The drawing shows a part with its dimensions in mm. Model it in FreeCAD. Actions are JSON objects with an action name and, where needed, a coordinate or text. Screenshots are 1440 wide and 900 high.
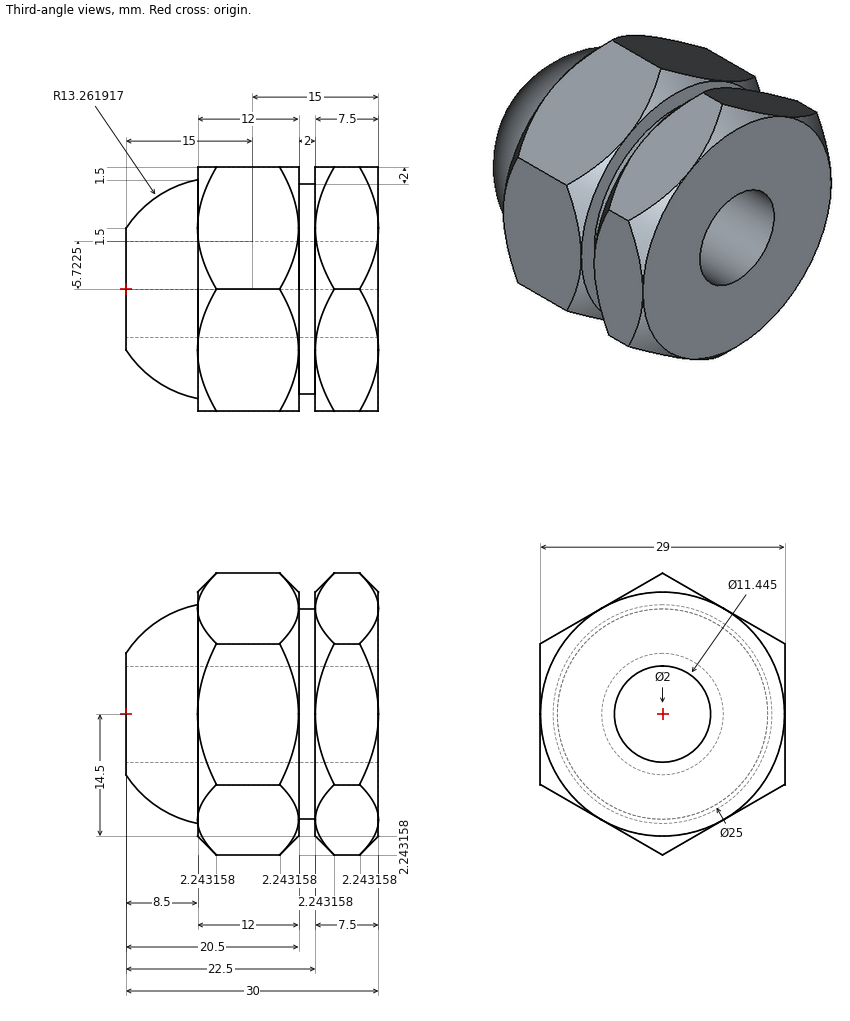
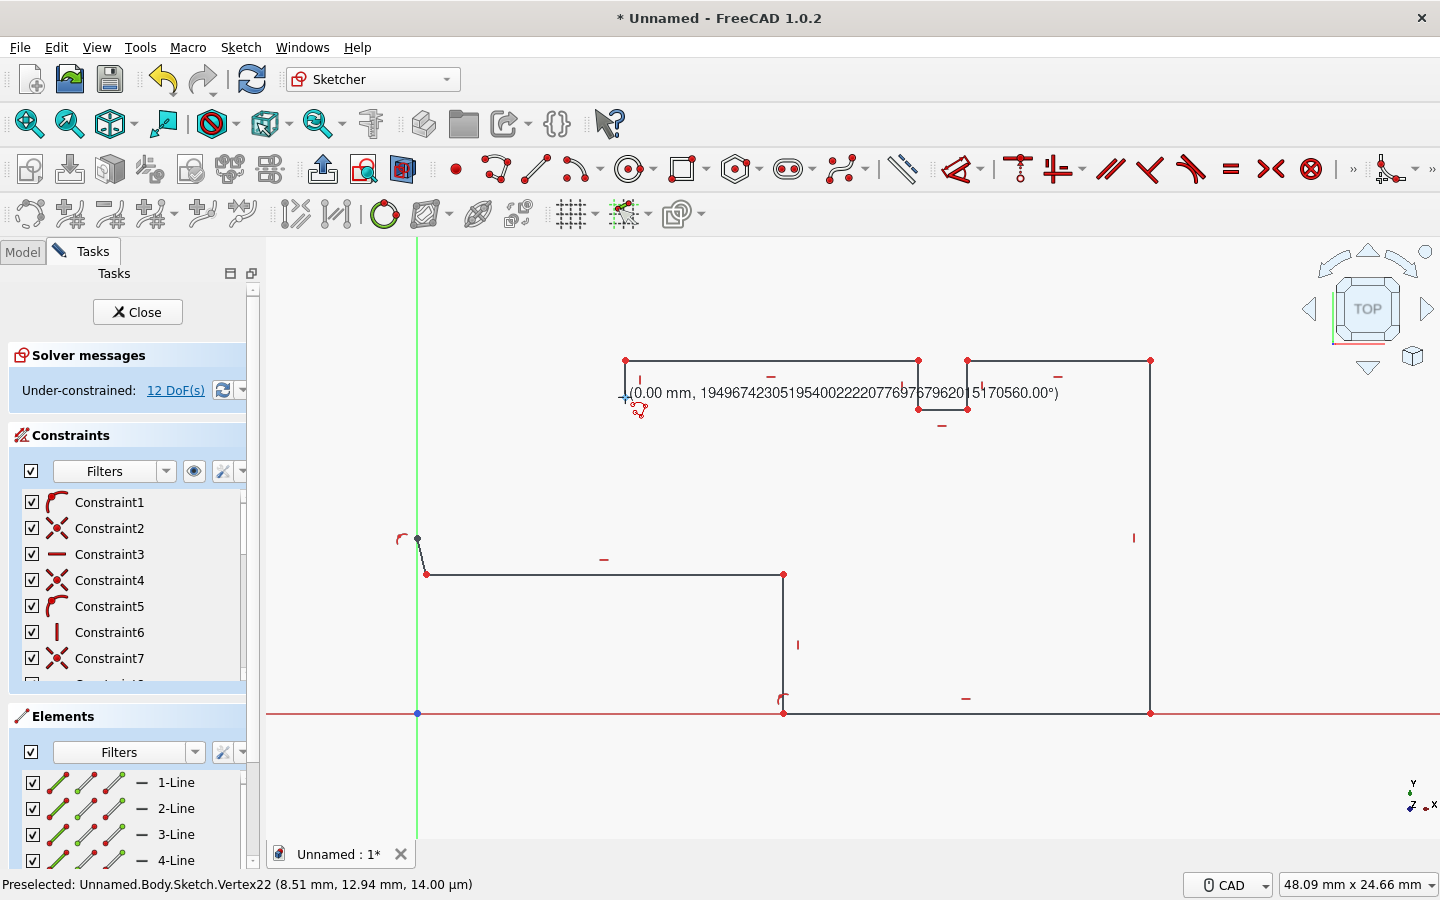
{"action": "left_click", "coordinate": [602, 170]}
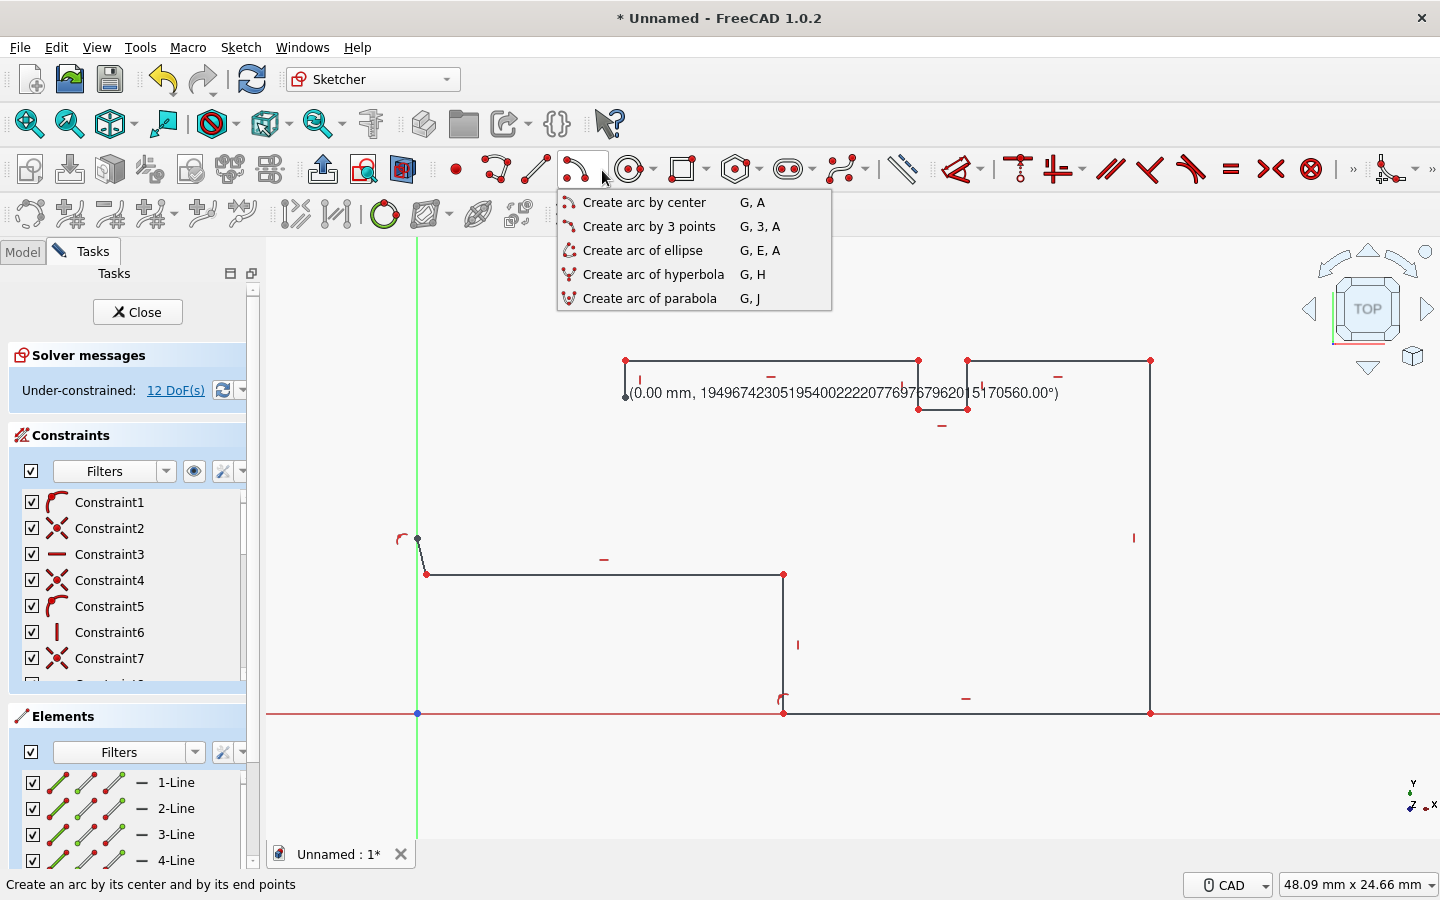
{"action": "left_click", "coordinate": [694, 226]}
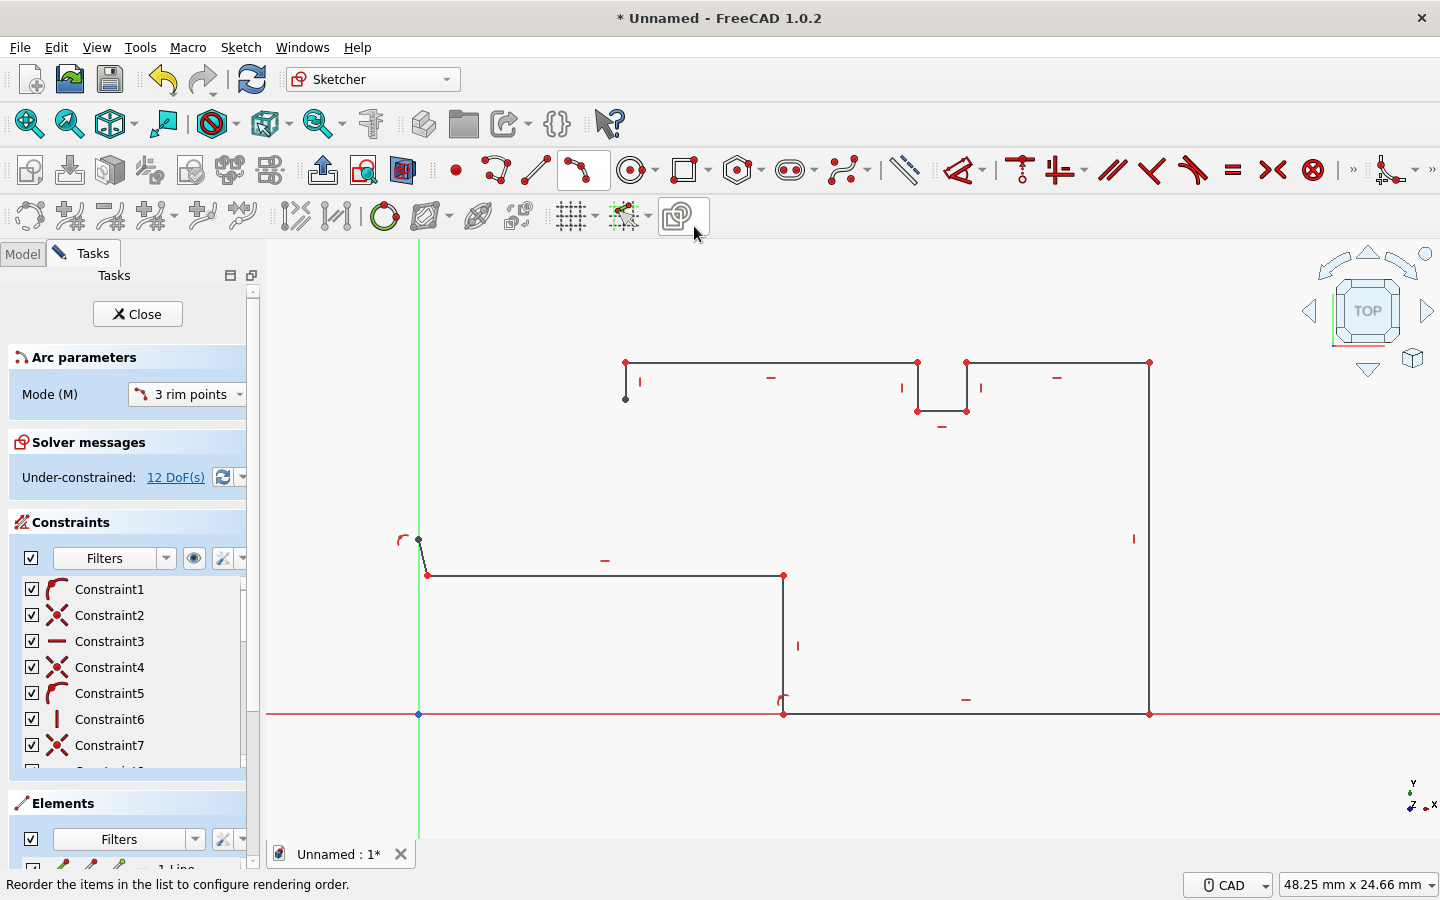
{"action": "left_click", "coordinate": [626, 399]}
{"action": "left_click", "coordinate": [419, 540]}
{"action": "left_click", "coordinate": [508, 448]}
{"action": "key", "text": "Escape"}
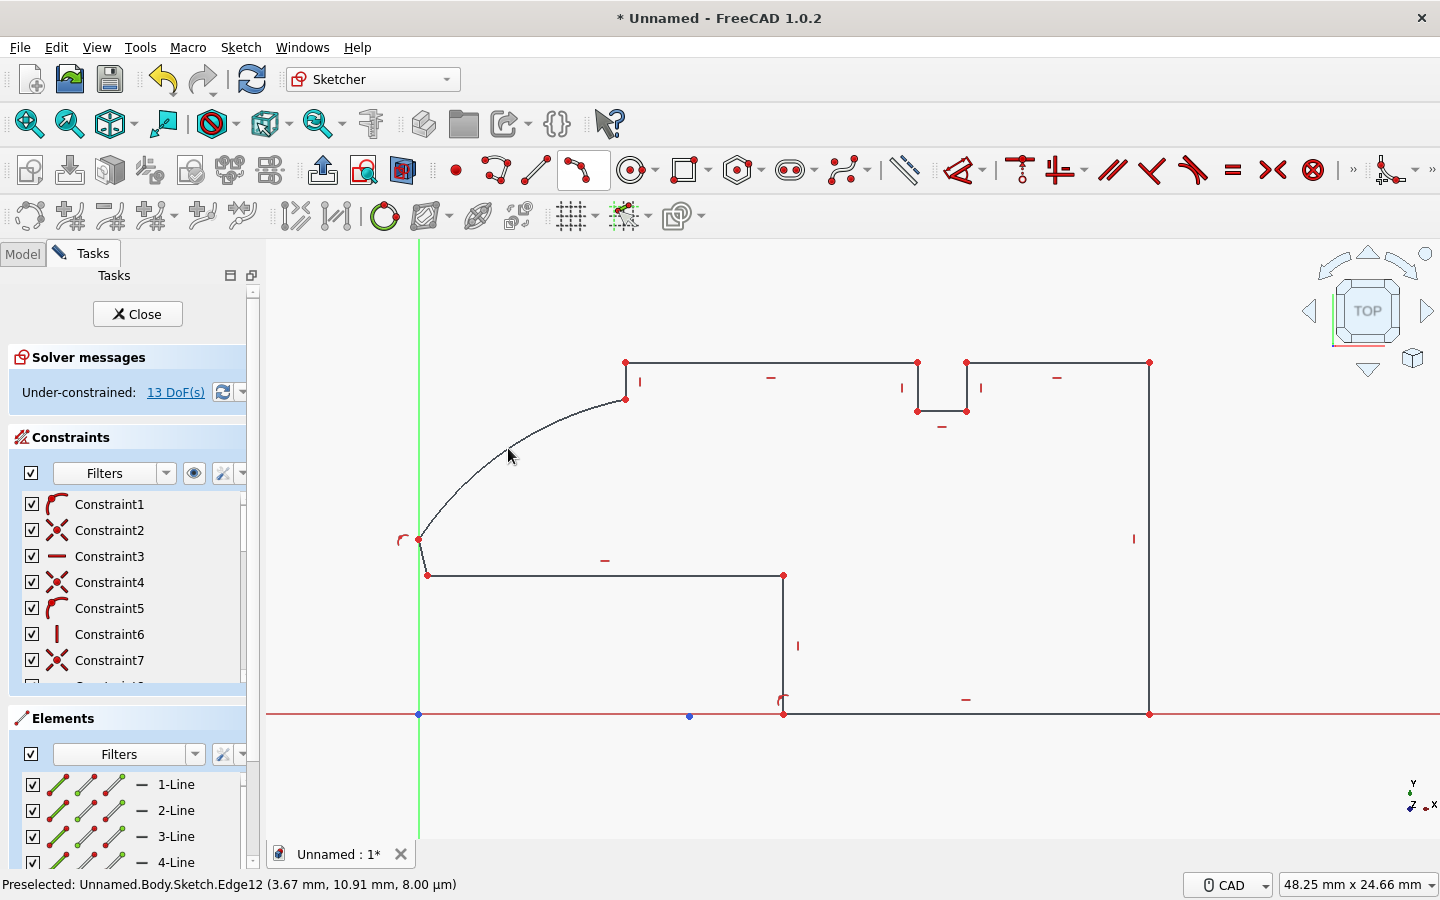
{"action": "scroll", "coordinate": [421, 551], "scroll_direction": "up", "scroll_amount": 2}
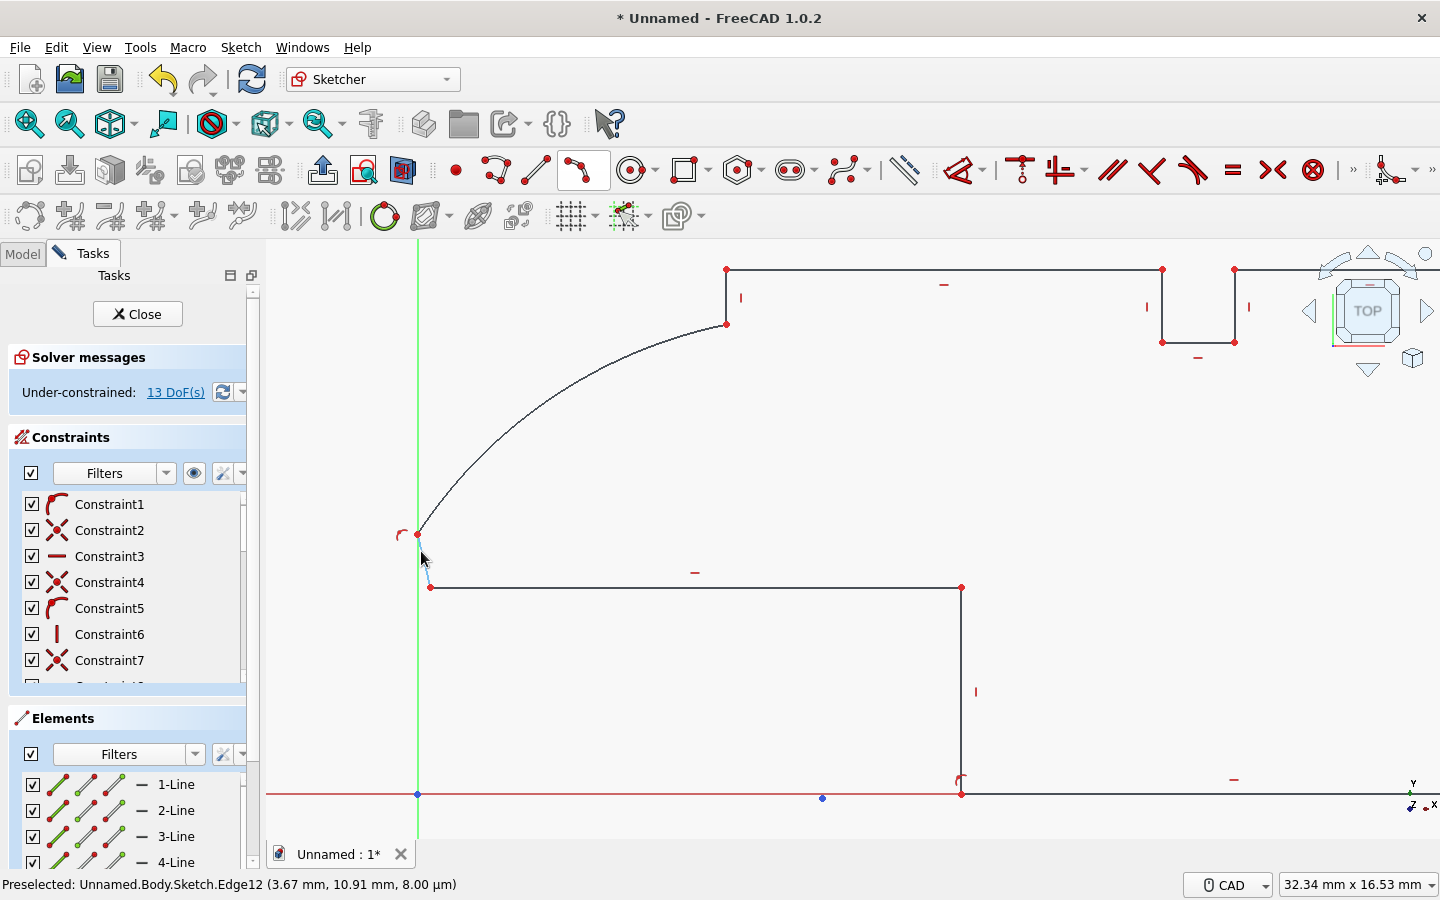
{"action": "left_click", "coordinate": [421, 550]}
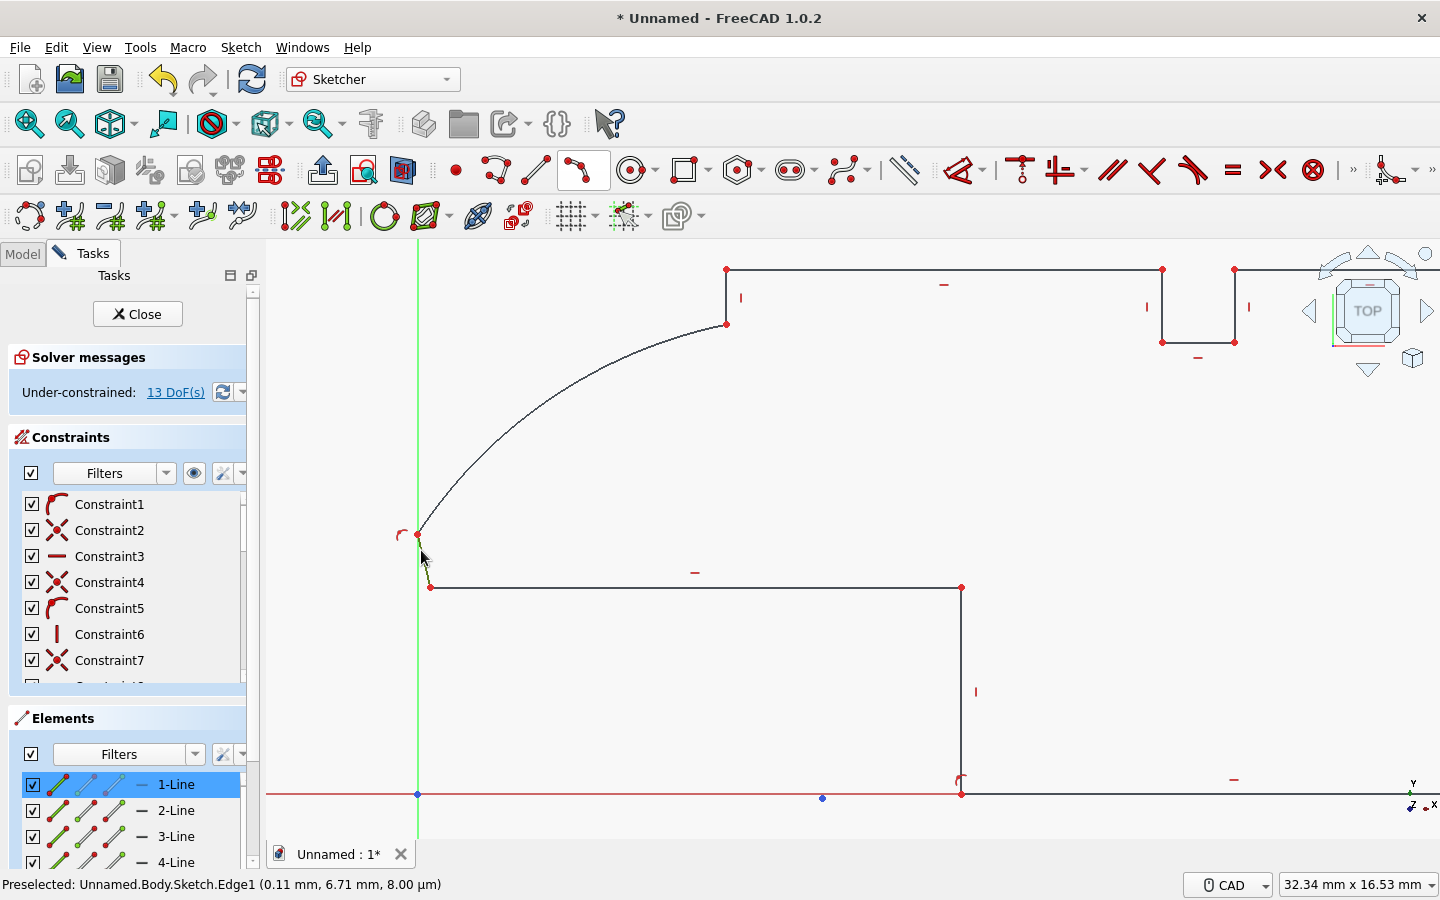
{"action": "key", "text": "v"}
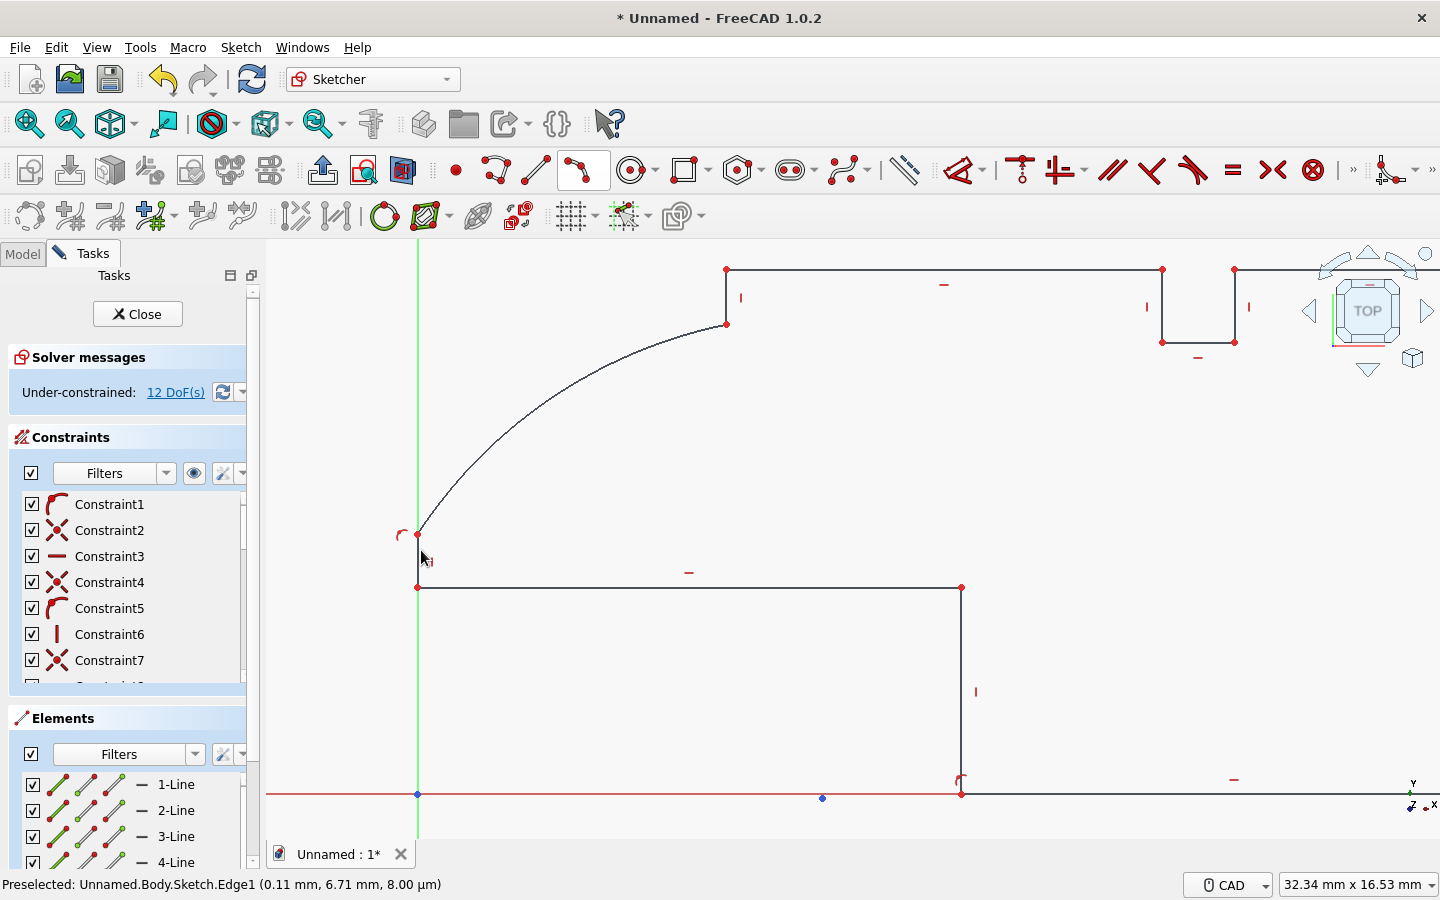
{"action": "left_click", "coordinate": [822, 798]}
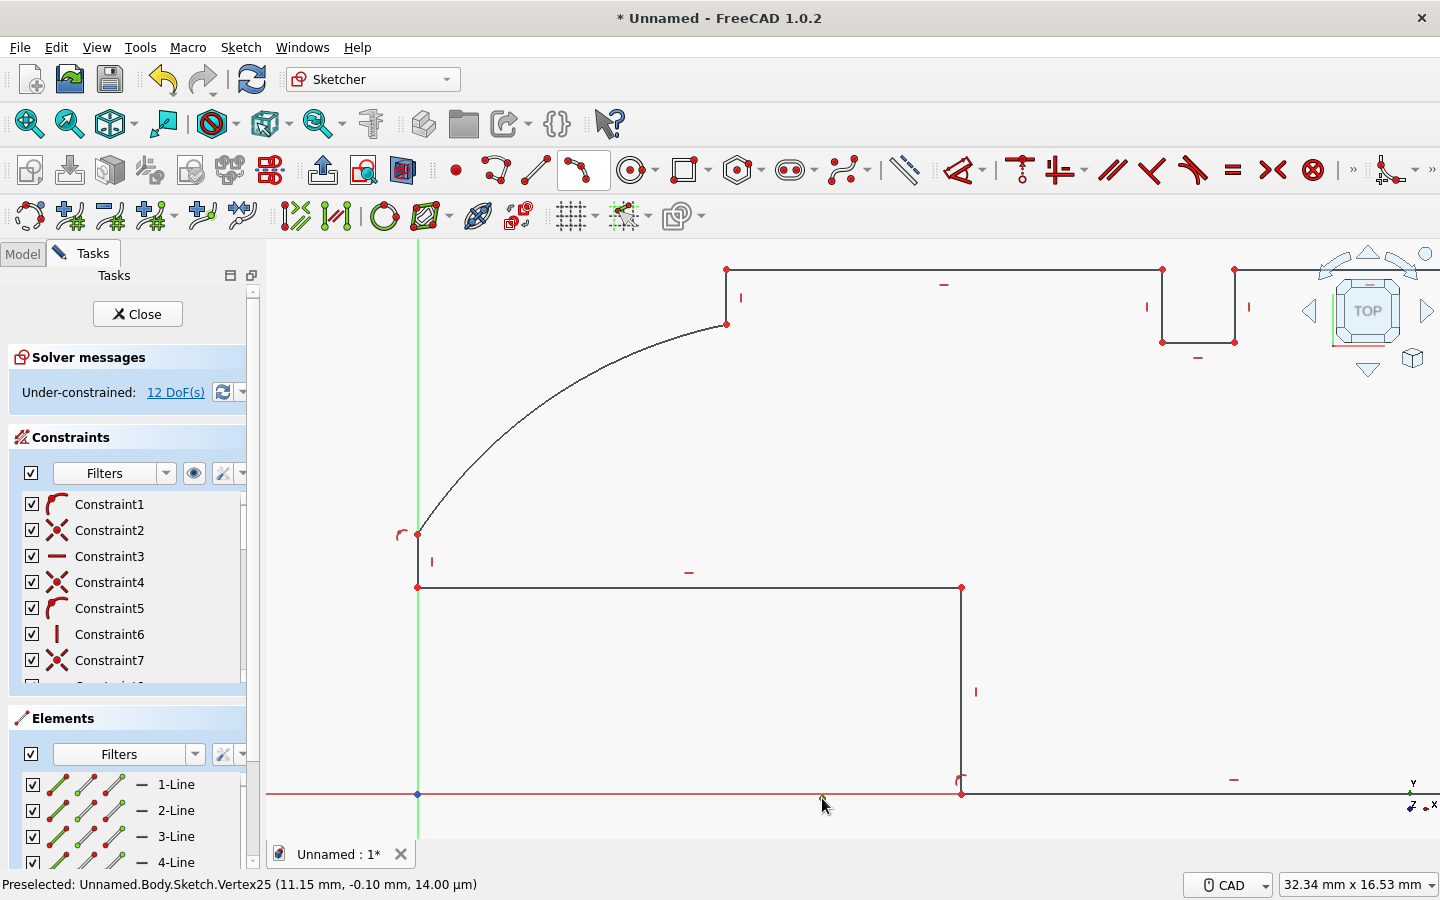
{"action": "left_click", "coordinate": [364, 794]}